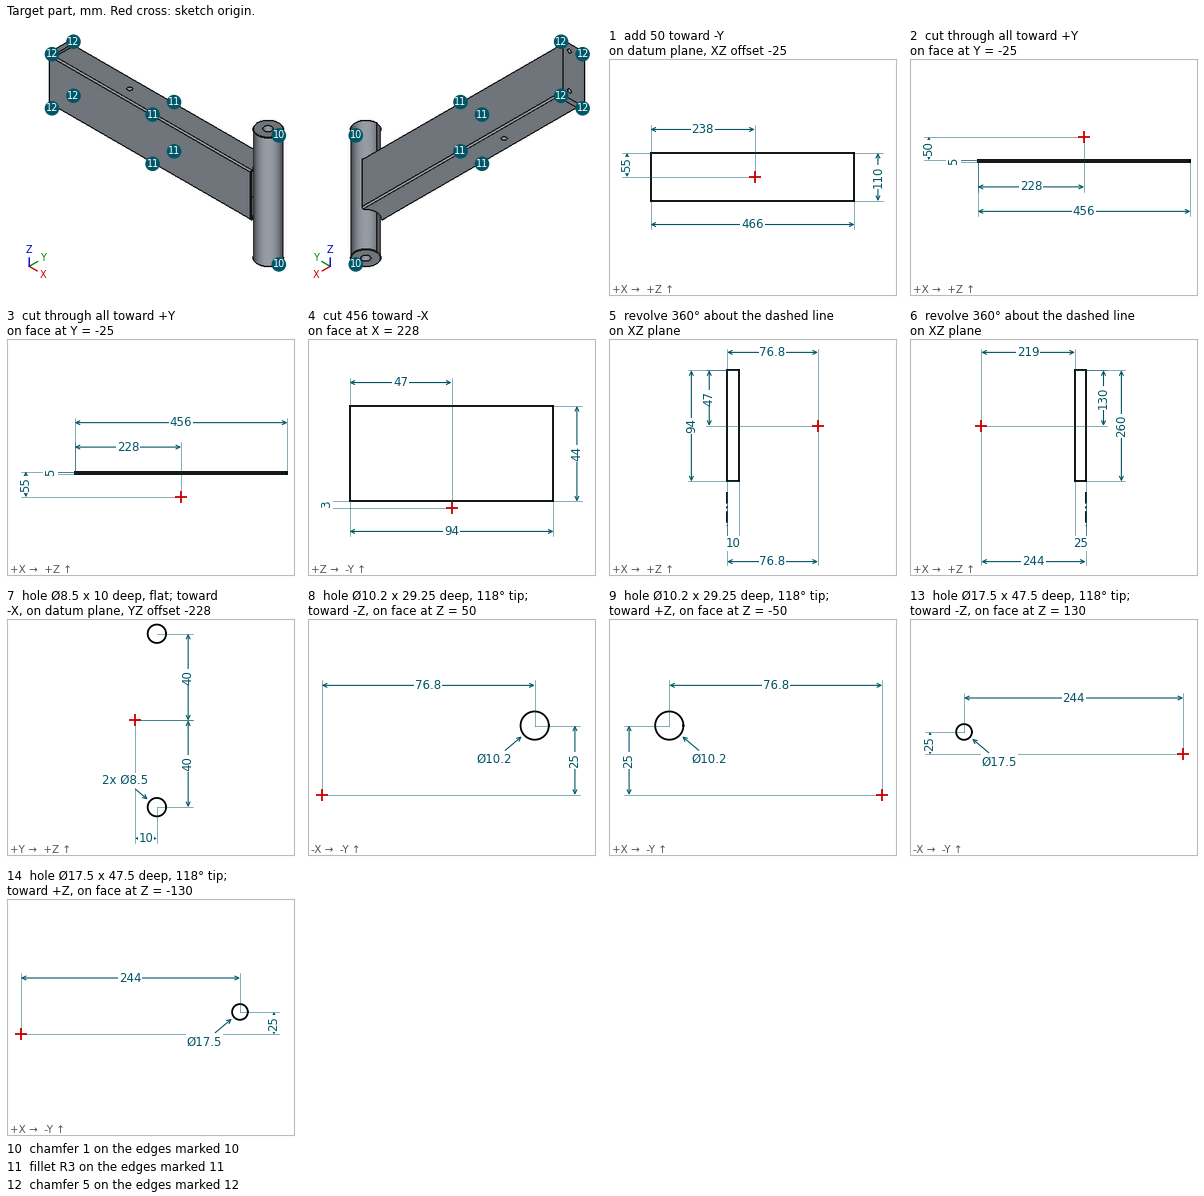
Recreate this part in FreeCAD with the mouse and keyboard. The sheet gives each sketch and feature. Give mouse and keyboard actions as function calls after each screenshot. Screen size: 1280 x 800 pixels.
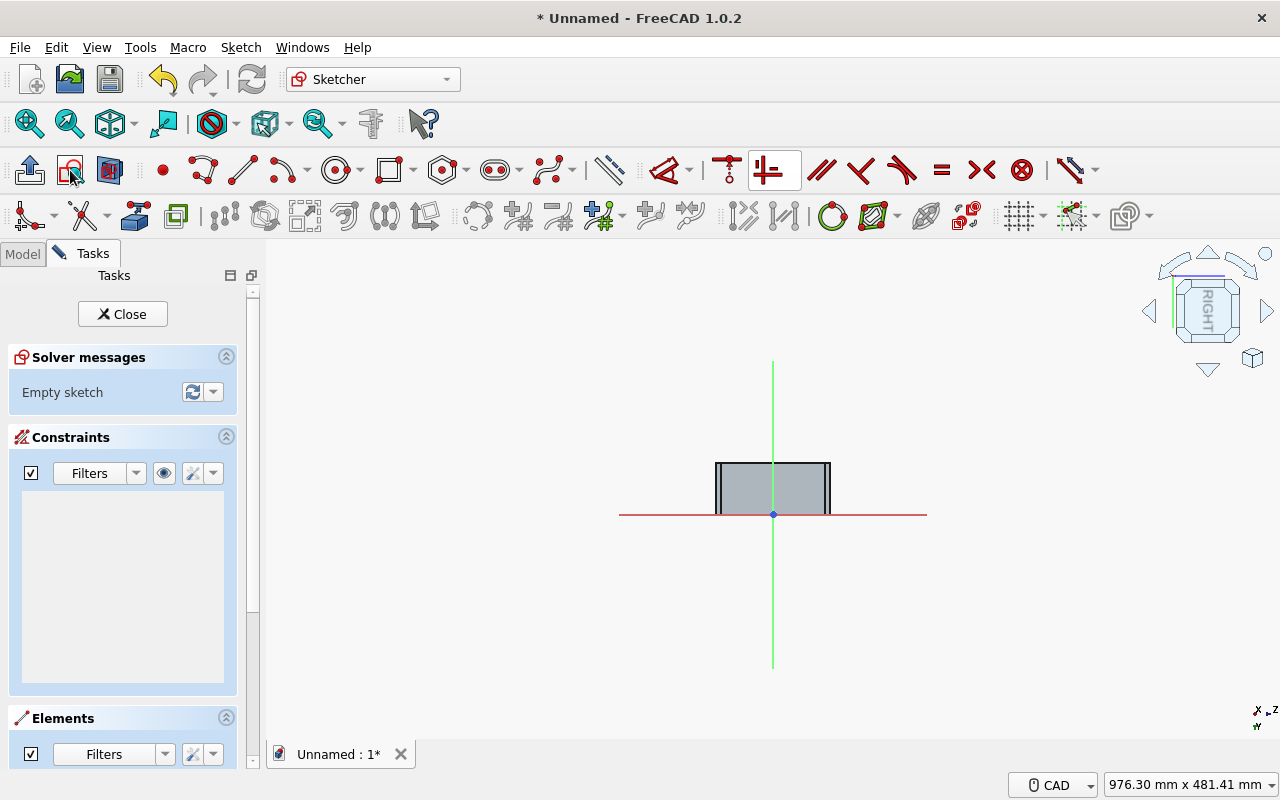
scroll(787, 491, up, 9)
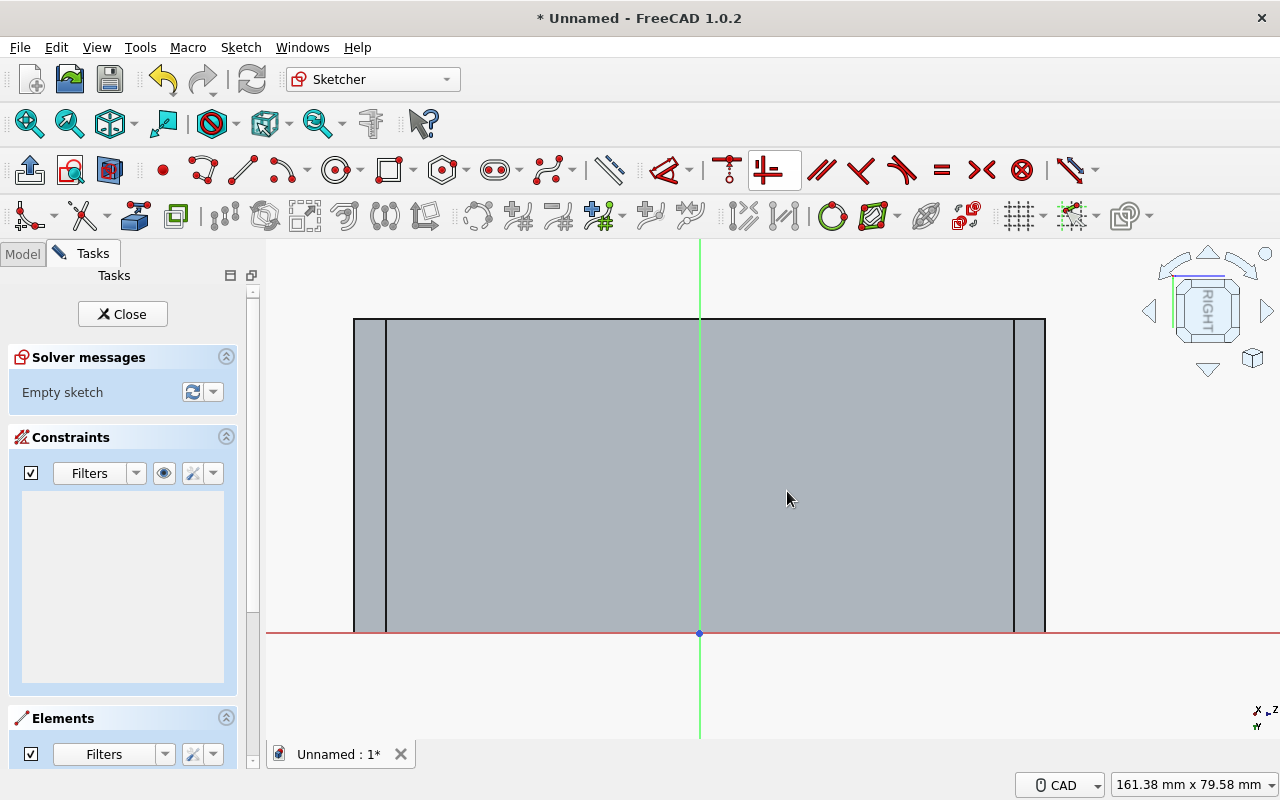
click(390, 170)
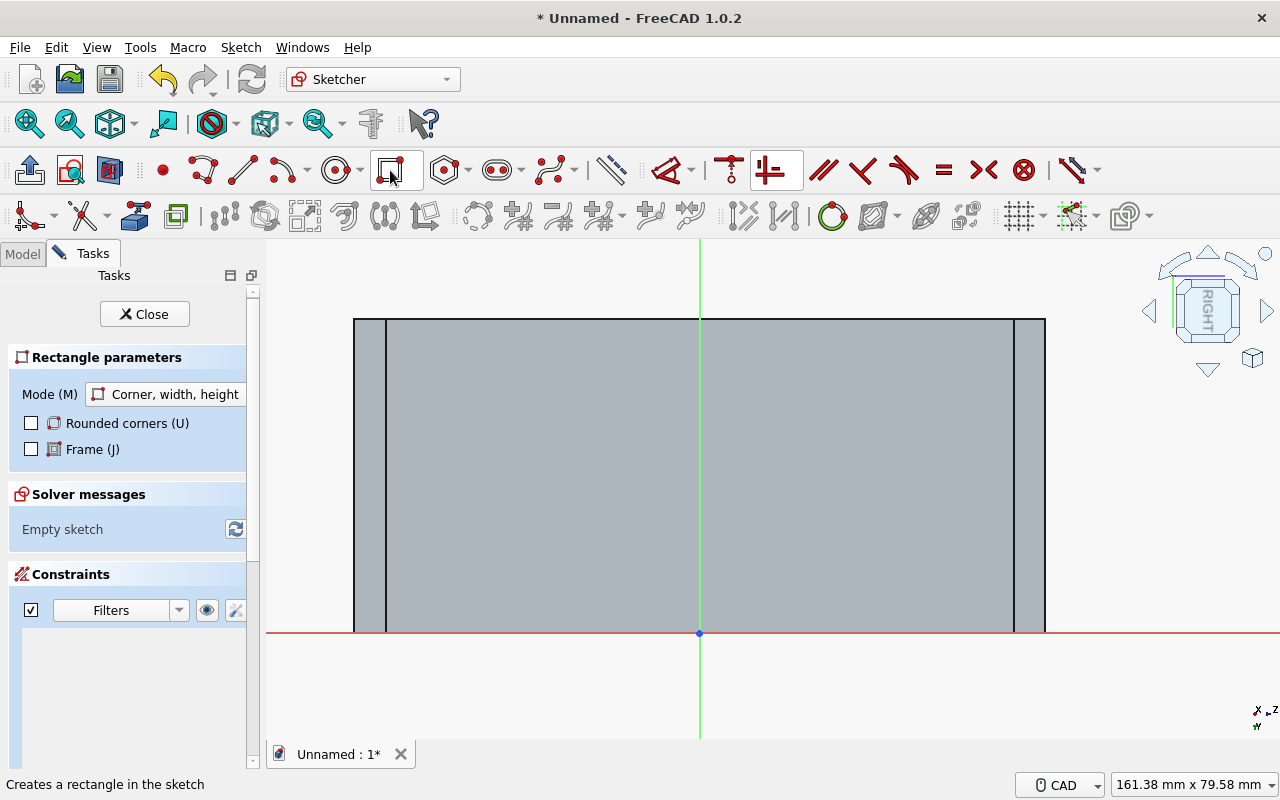
click(404, 338)
move(995, 615)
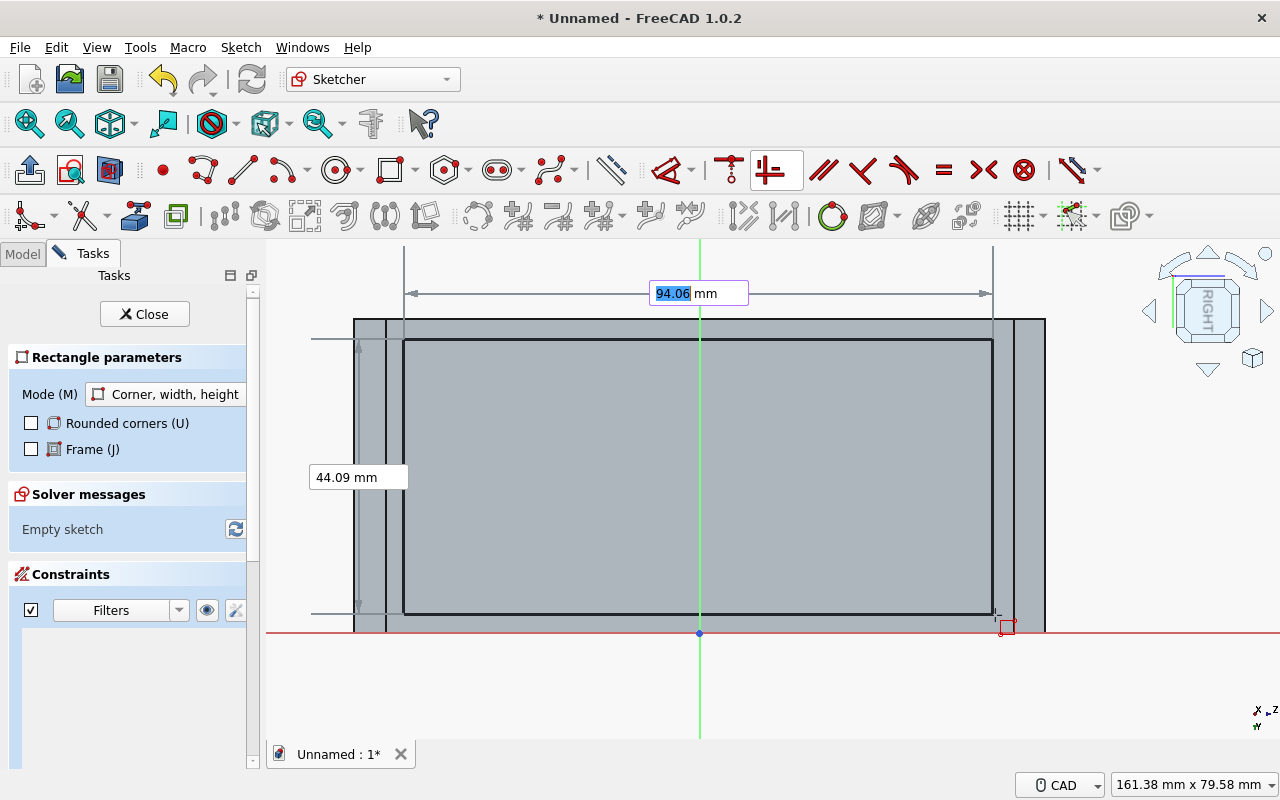
text(94)
key(Tab)
text(44)
key(Return)
key(Escape)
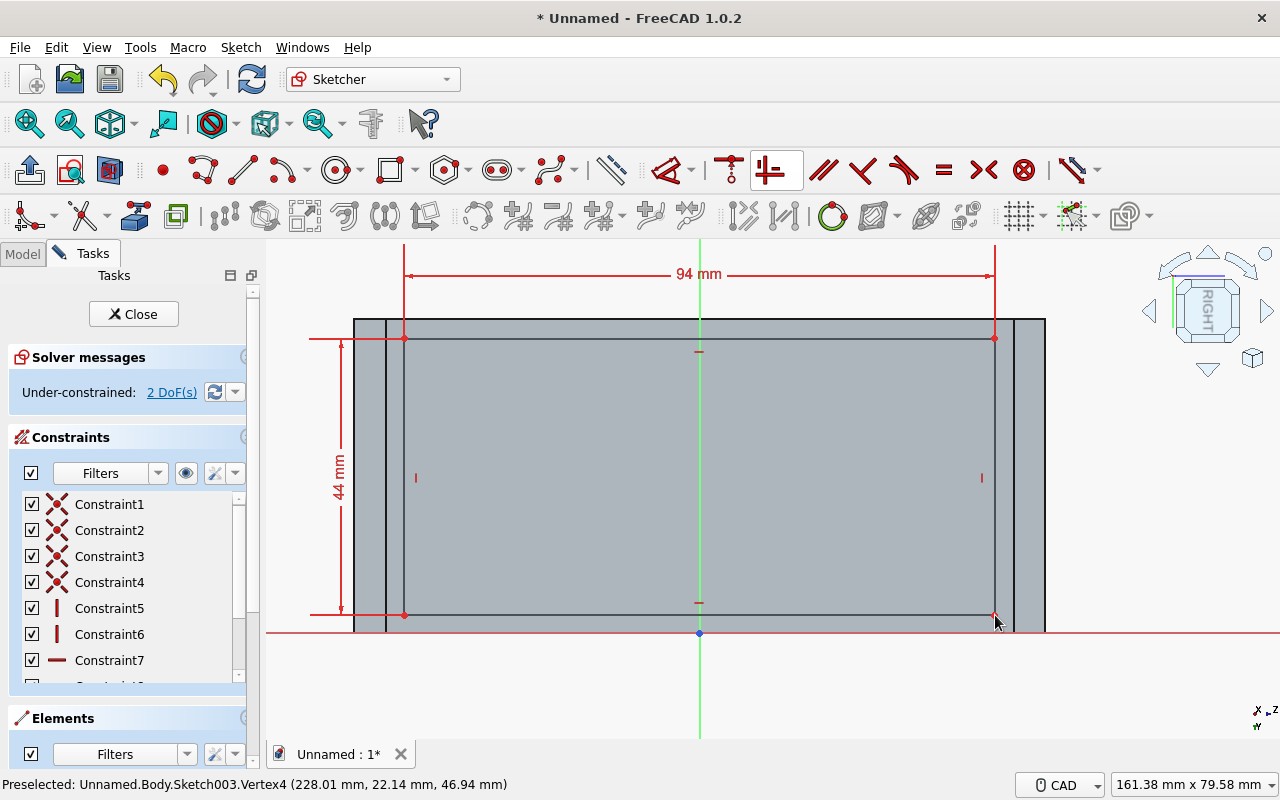
click(666, 170)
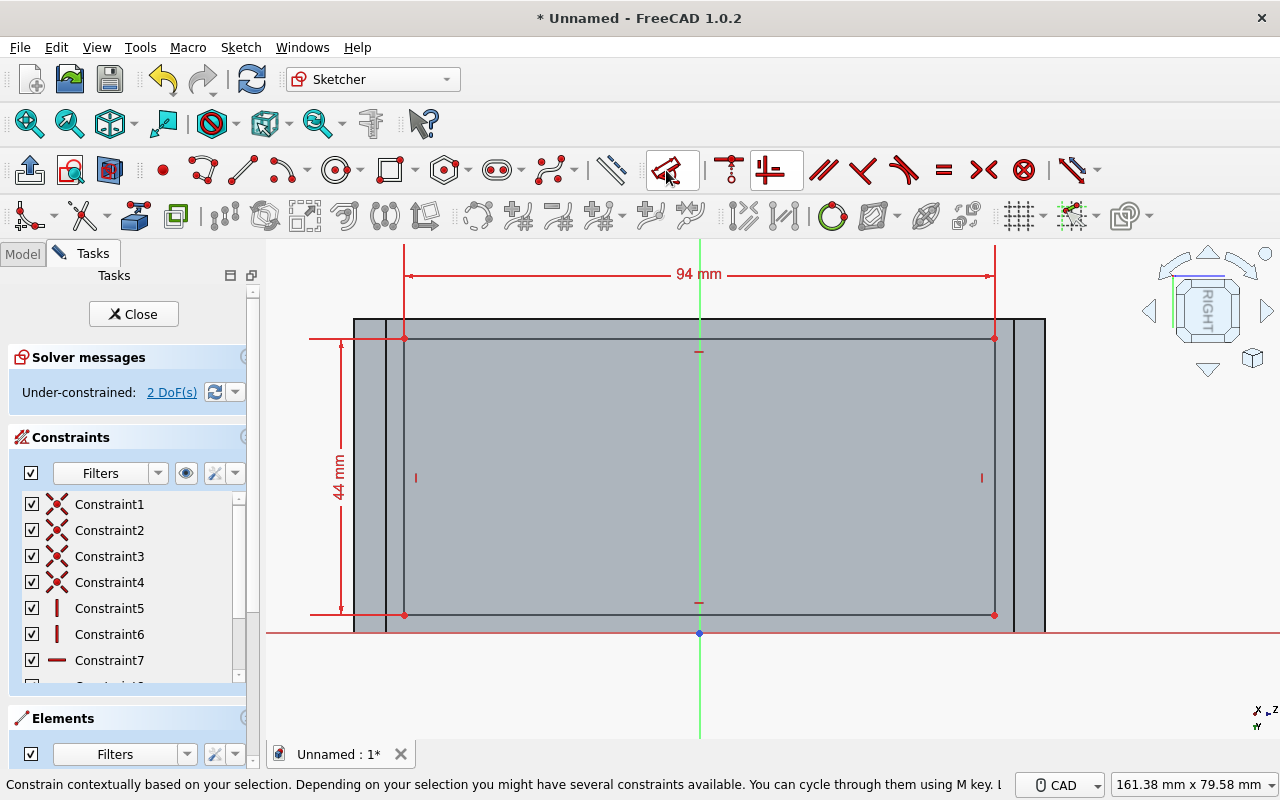
scroll(404, 615, up, 4)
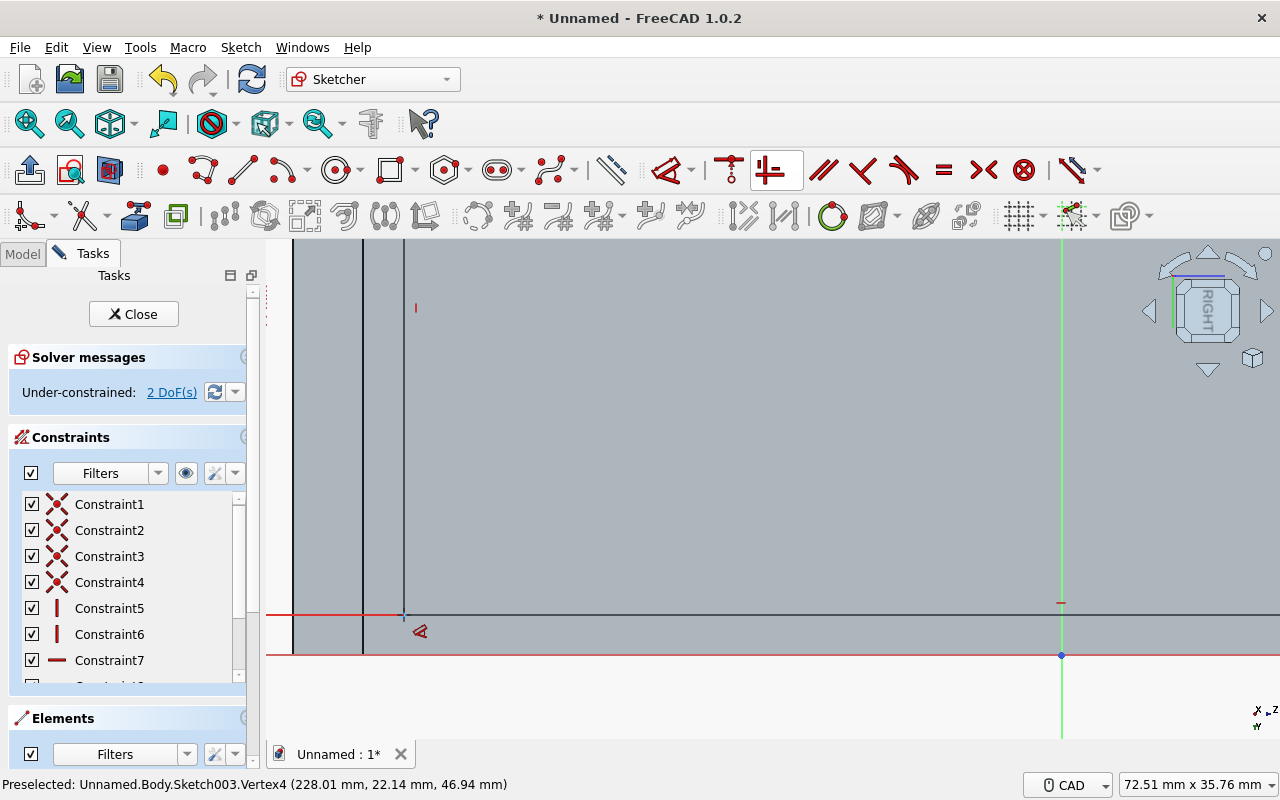
click(404, 615)
click(370, 635)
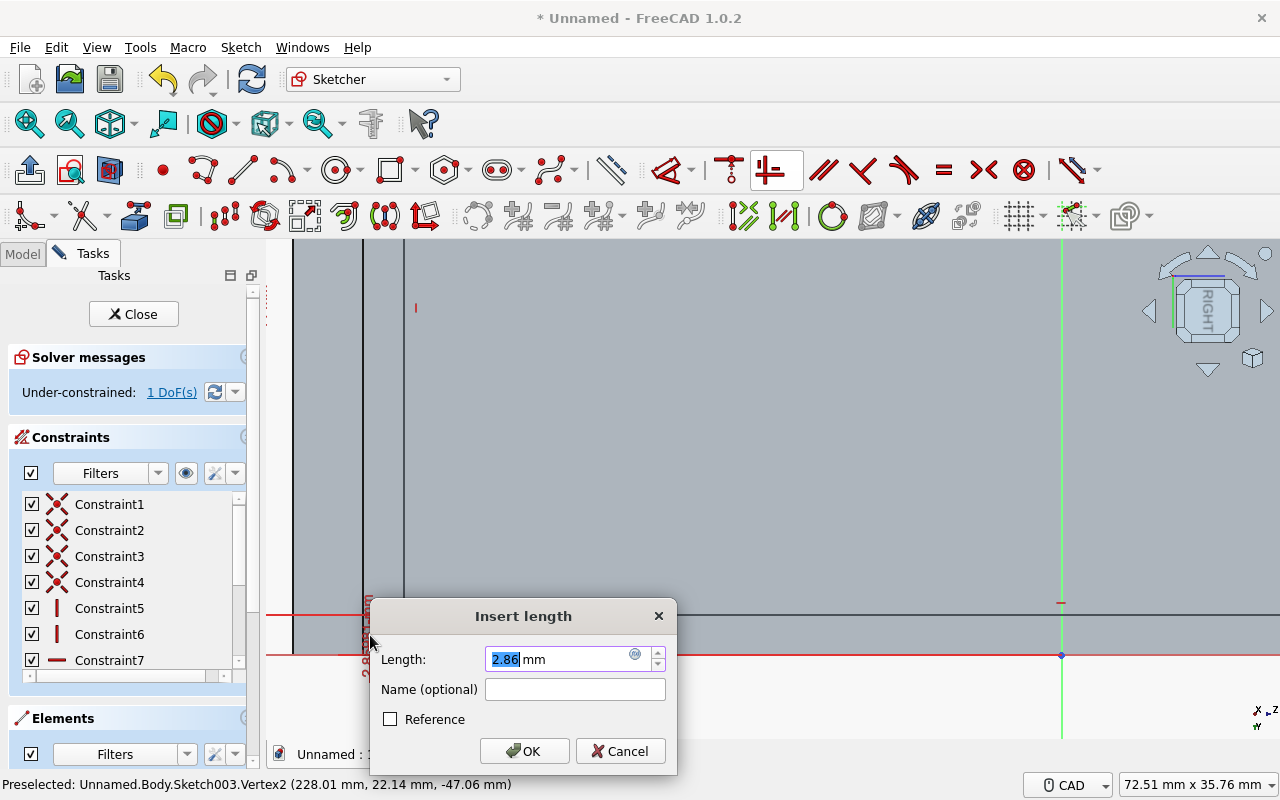
text(3)
key(Return)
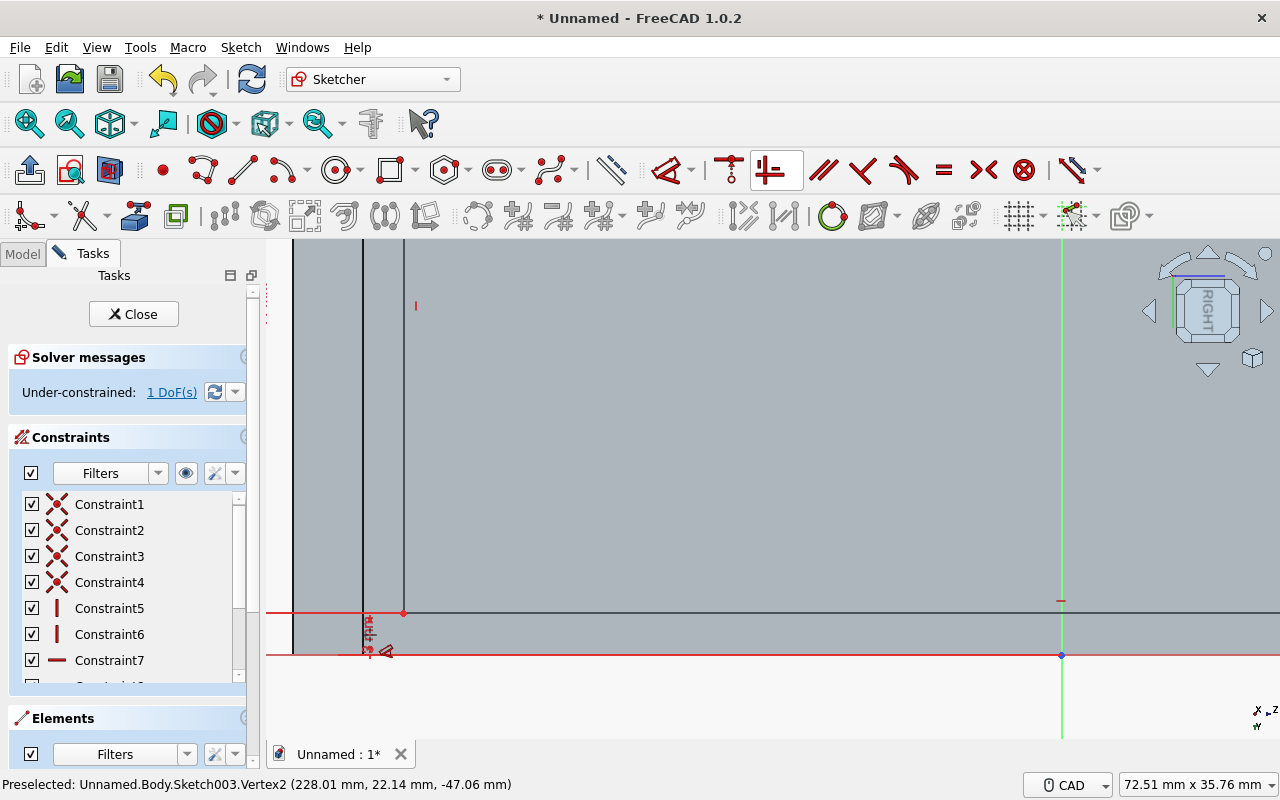
scroll(413, 622, down, 4)